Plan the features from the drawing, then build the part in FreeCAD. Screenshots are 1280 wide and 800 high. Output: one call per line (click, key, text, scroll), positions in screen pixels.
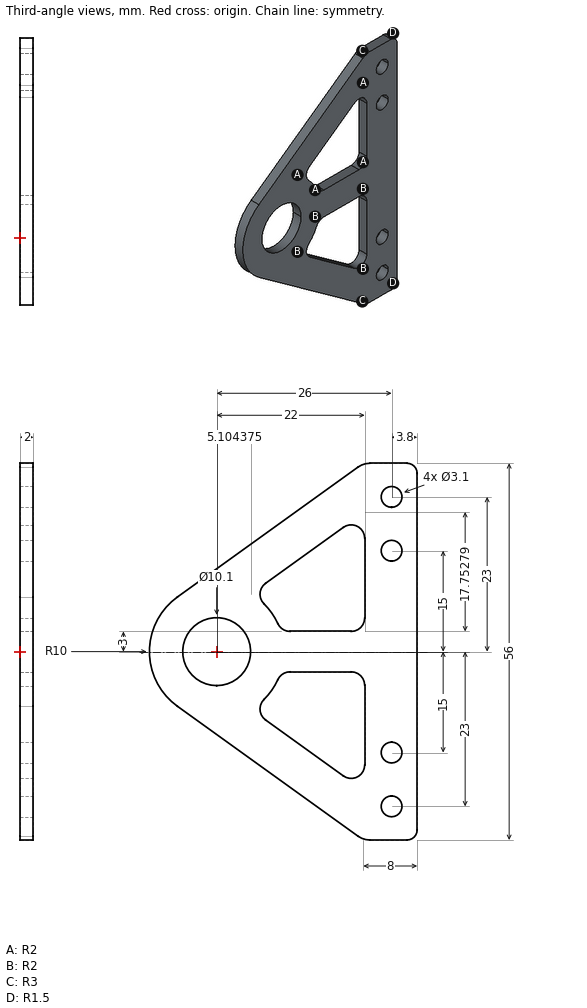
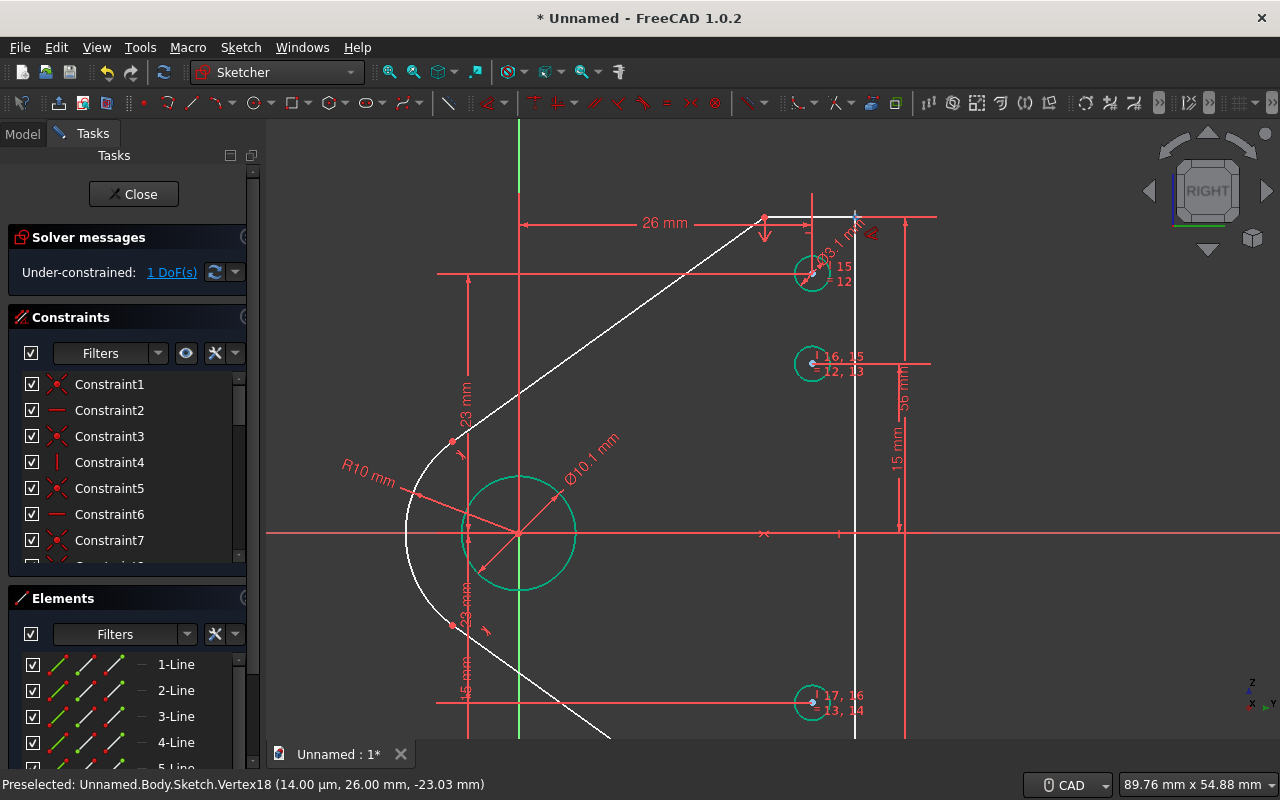
click(855, 217)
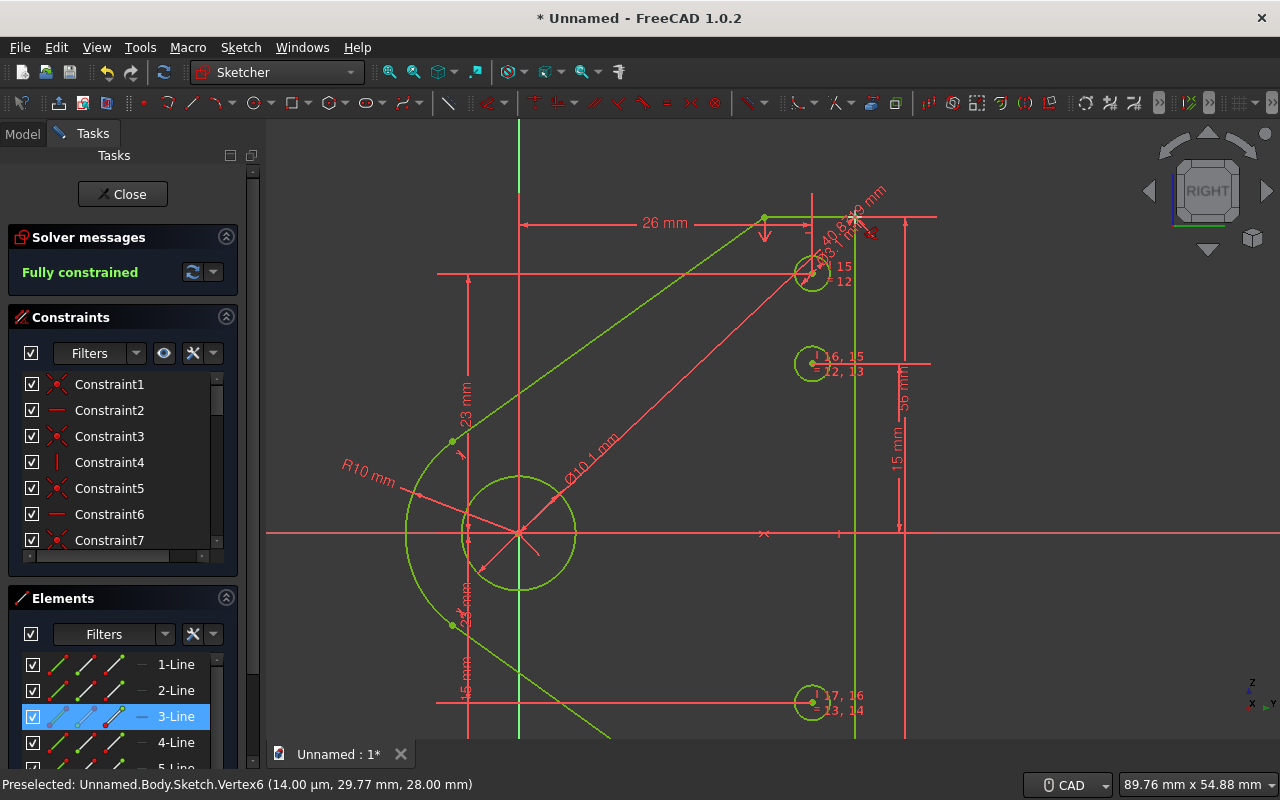
click(812, 274)
click(834, 183)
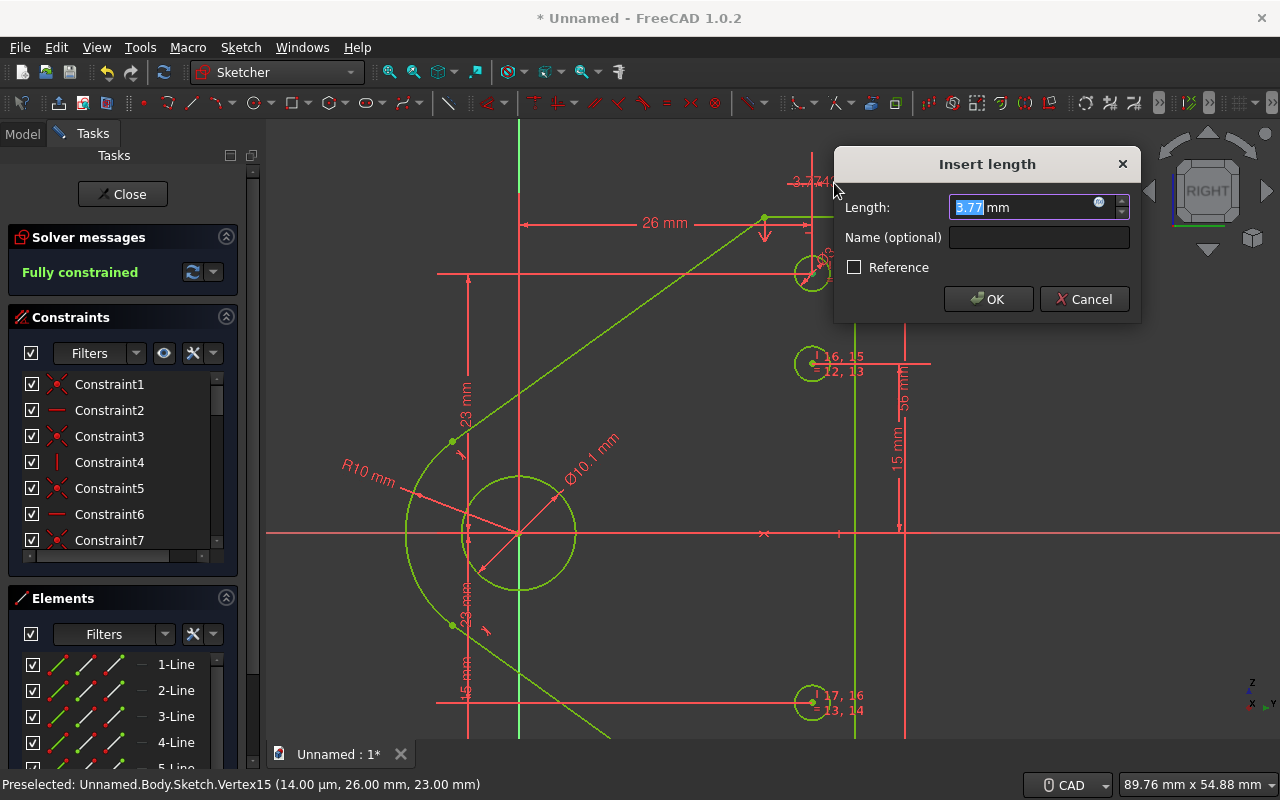
text(3.8)
key(Return)
key(Escape)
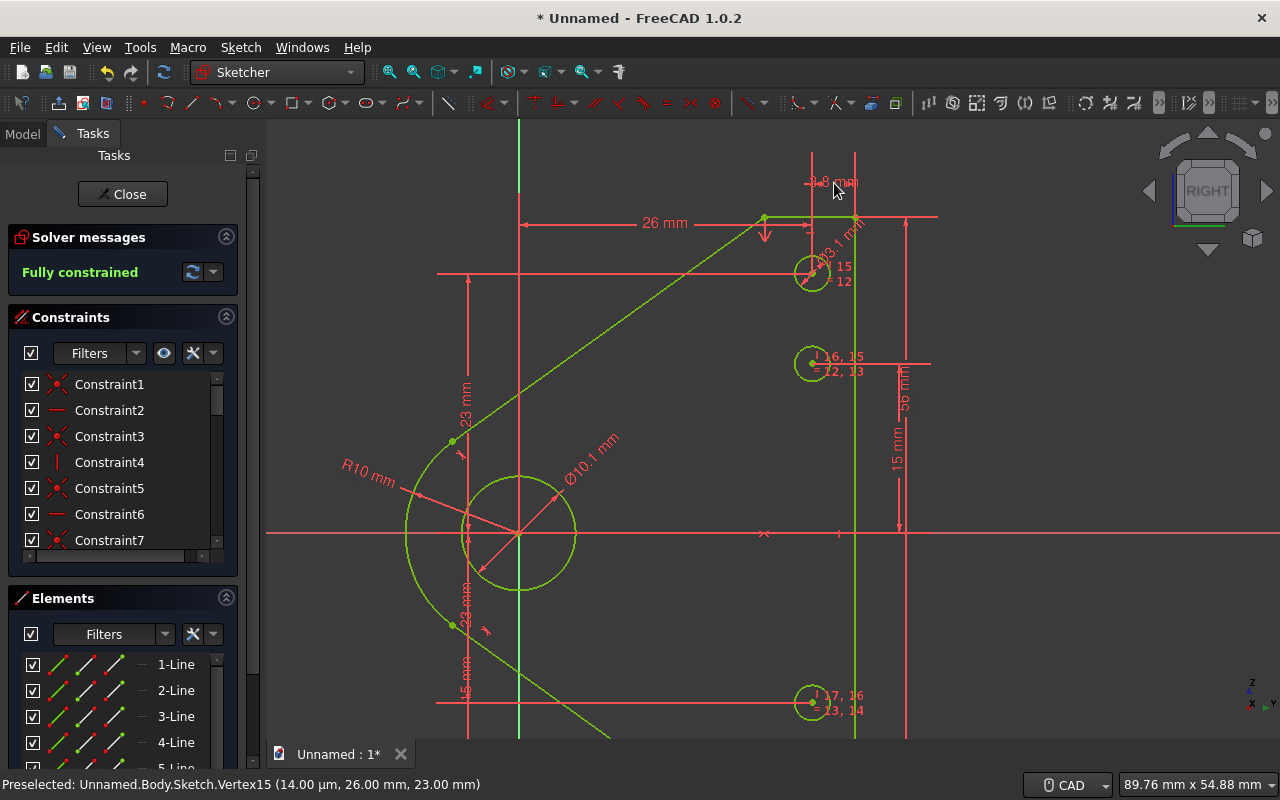
click(123, 194)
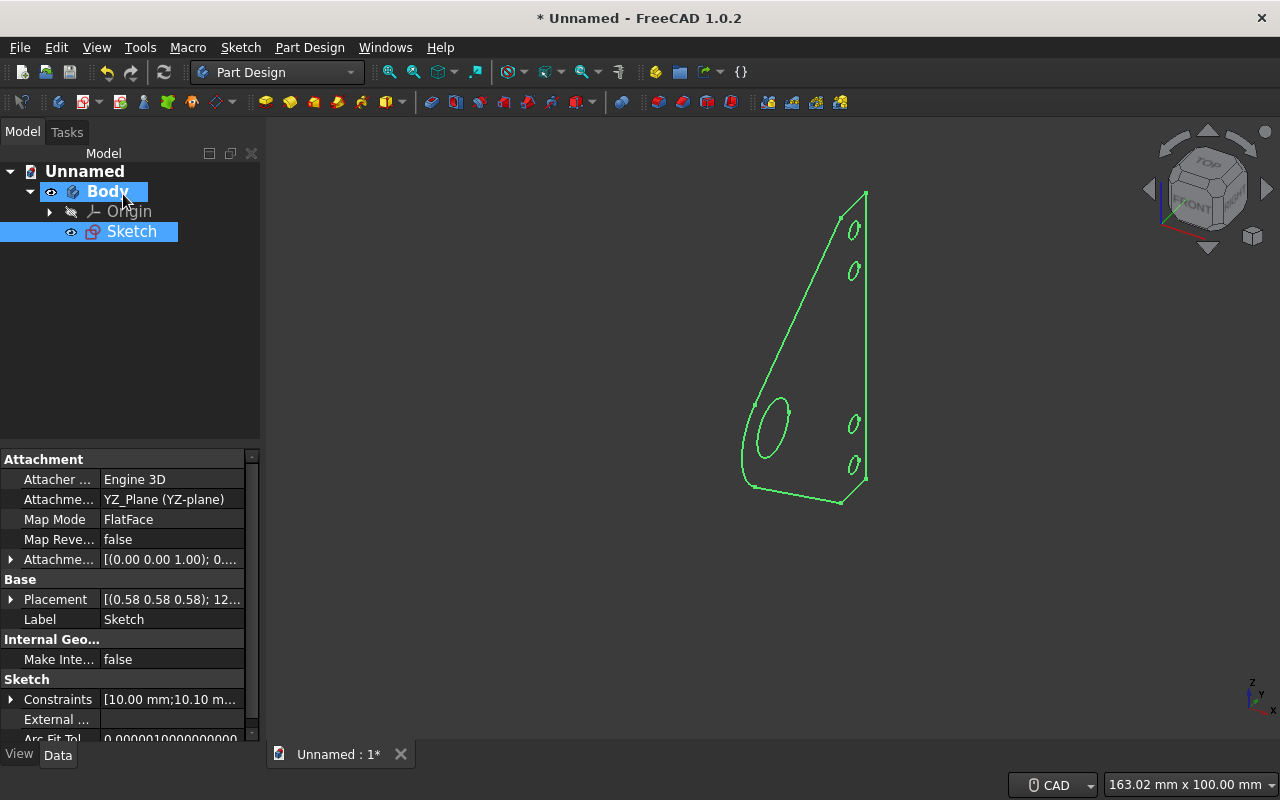
click(266, 102)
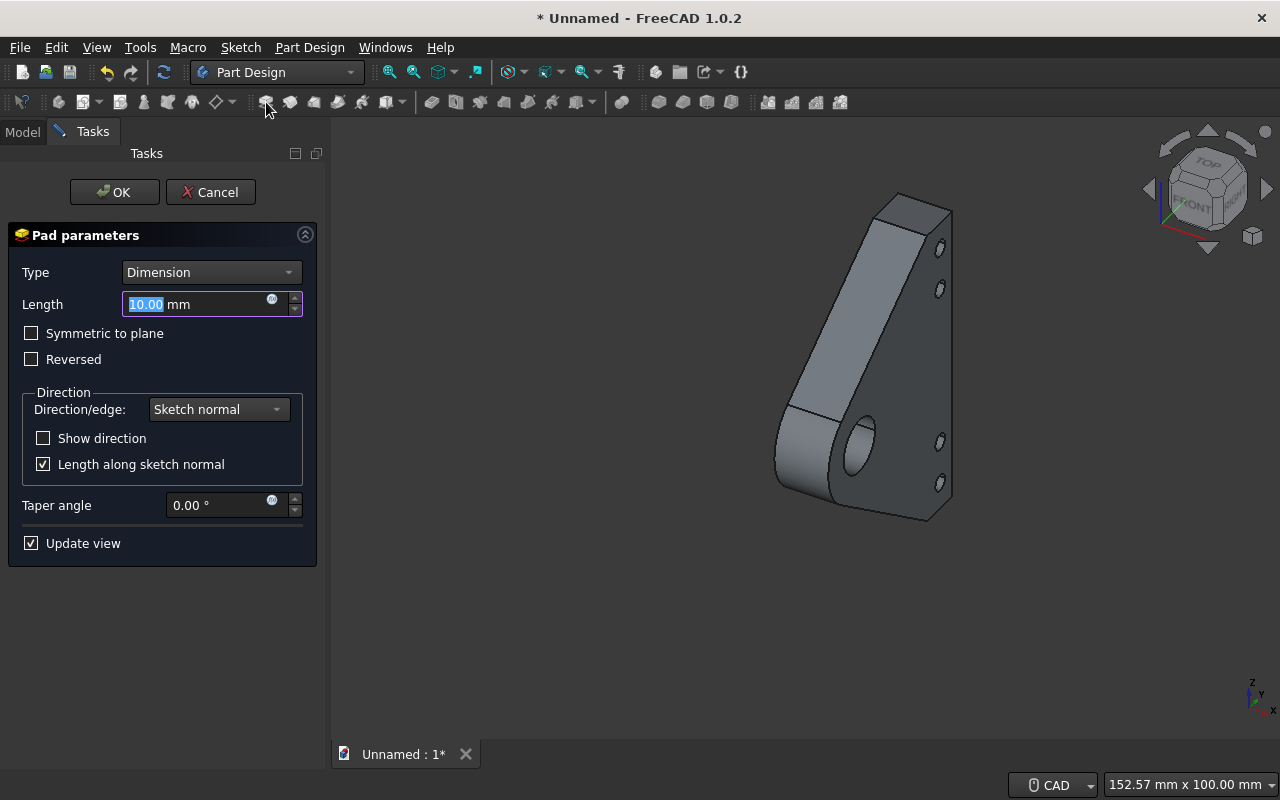
text(2)
key(Tab)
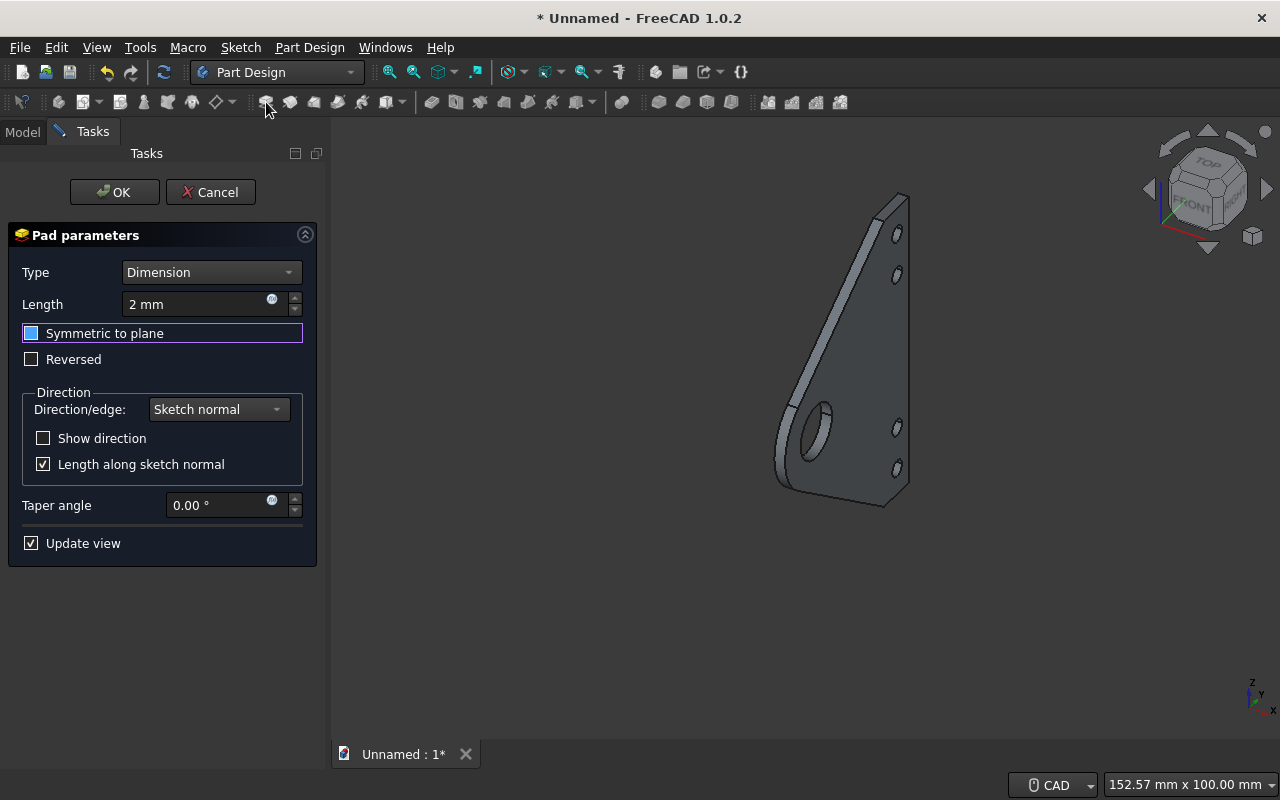
click(115, 192)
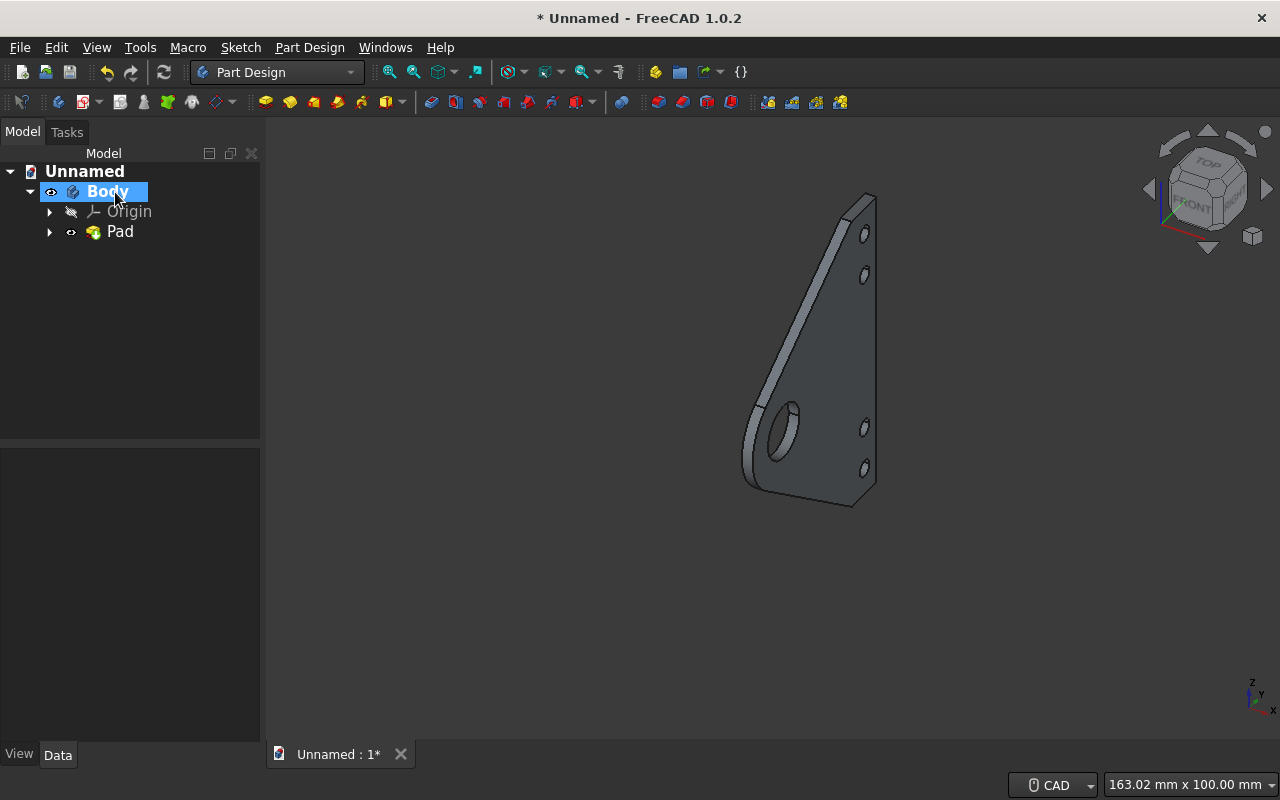
click(84, 102)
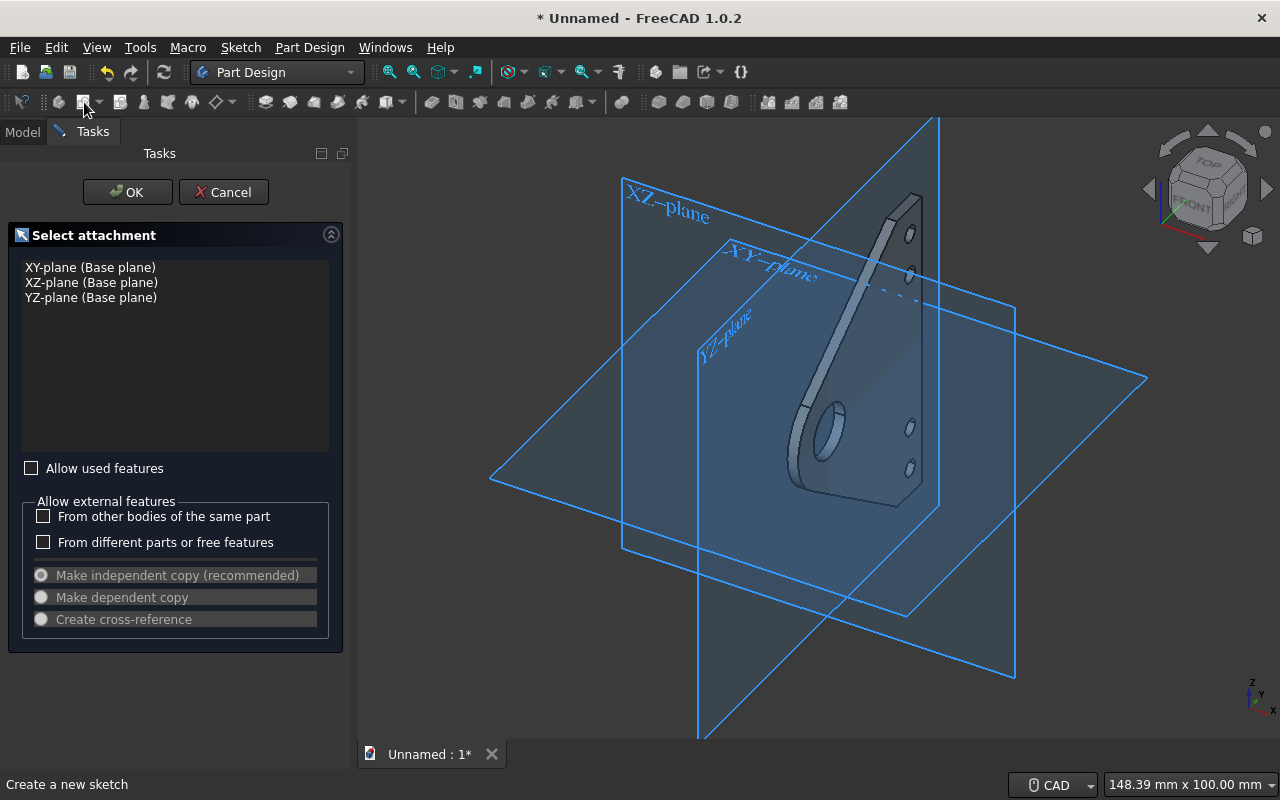
click(82, 298)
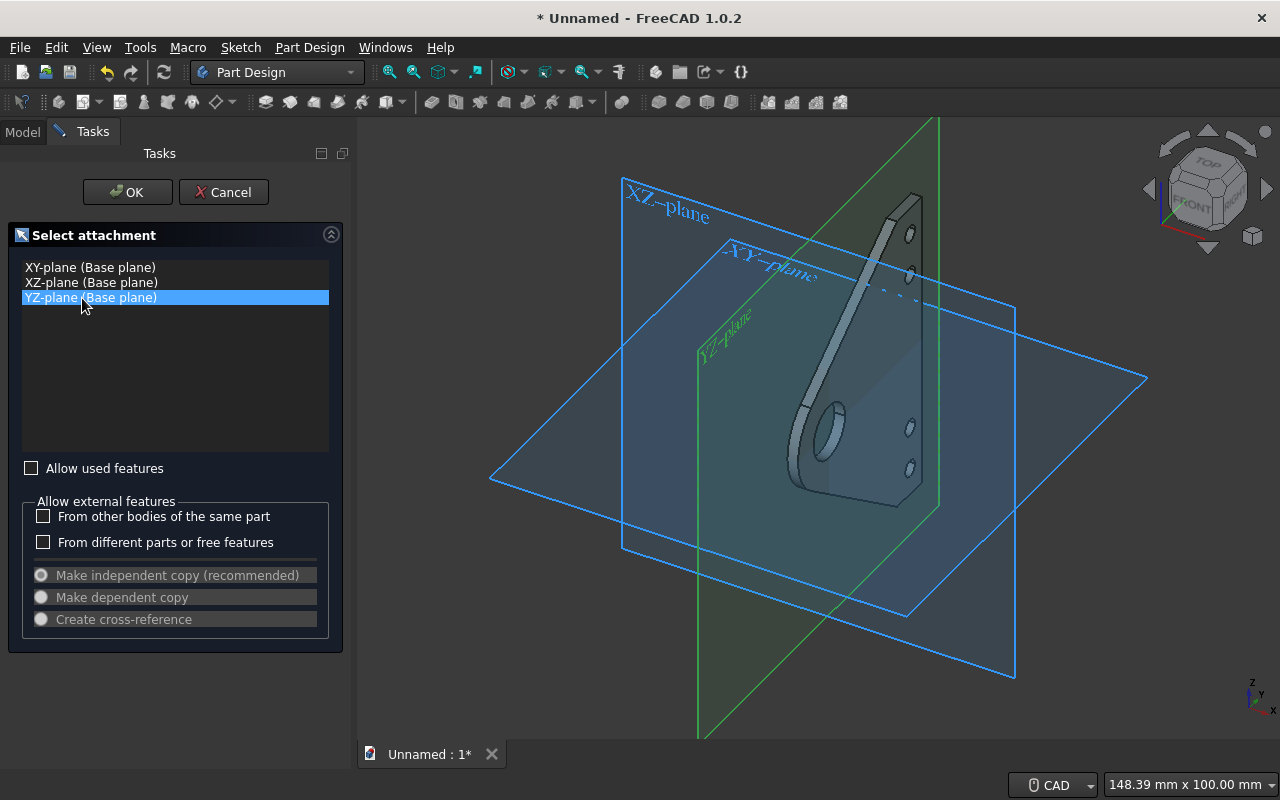
click(128, 192)